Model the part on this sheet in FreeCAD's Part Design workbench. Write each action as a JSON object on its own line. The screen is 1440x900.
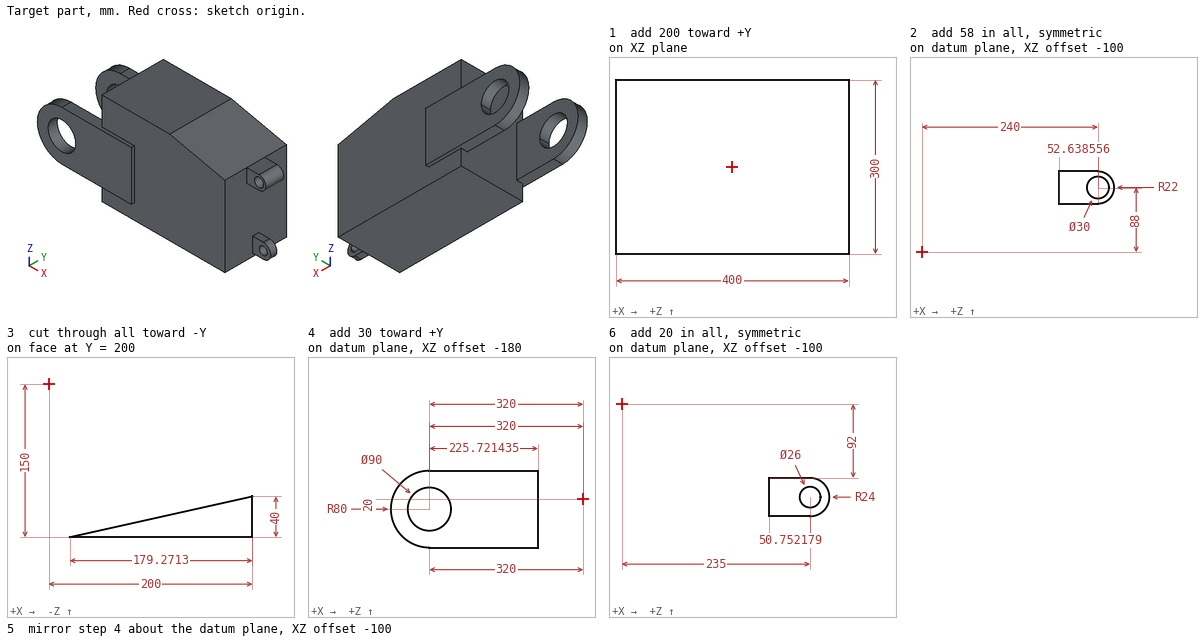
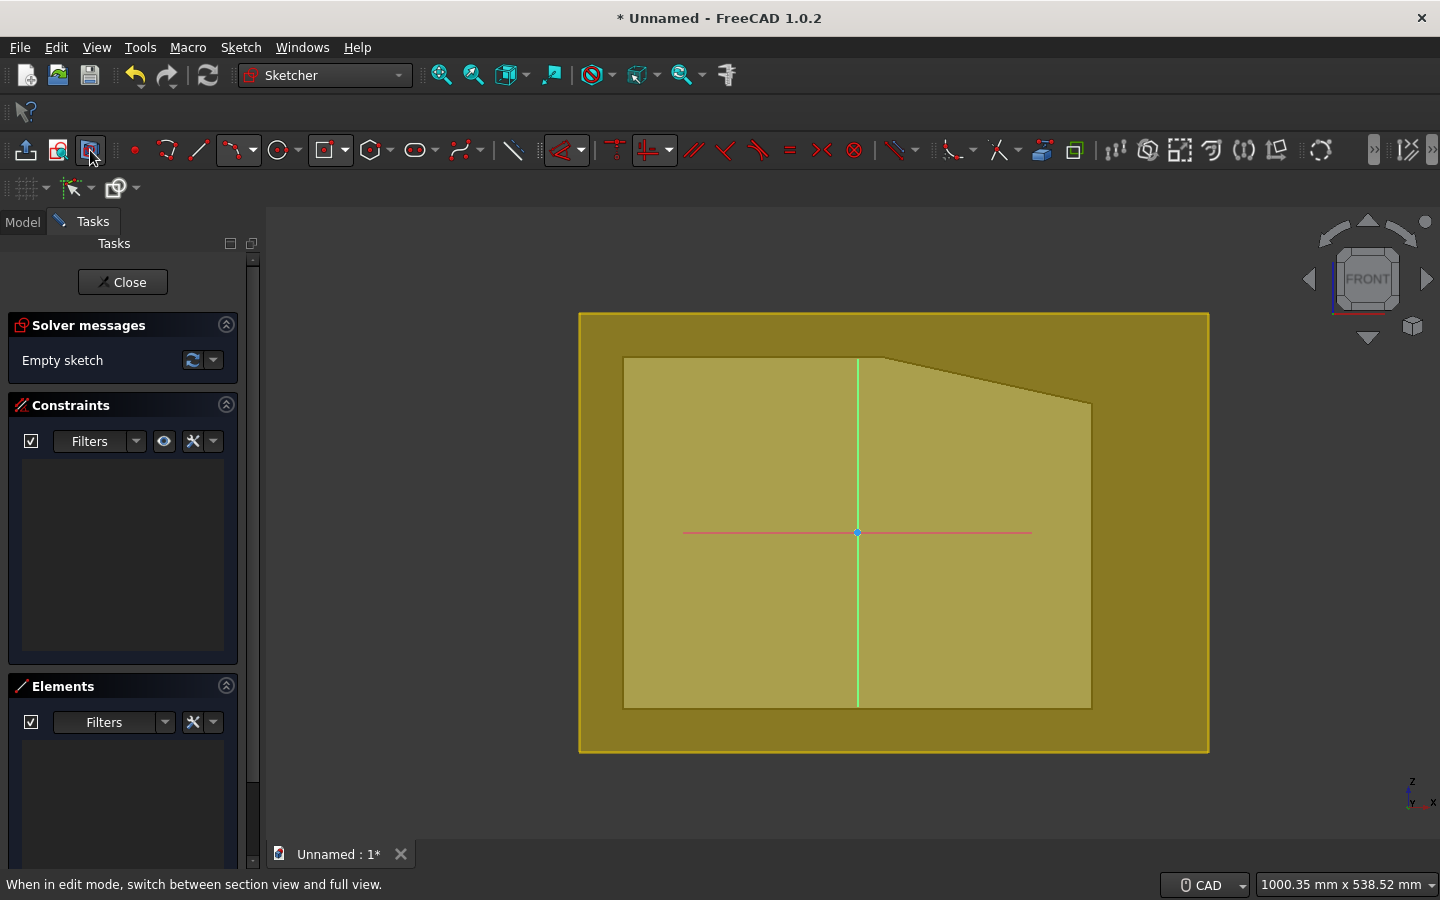
{"action": "scroll", "coordinate": [295, 624], "scroll_direction": "up", "scroll_amount": 2}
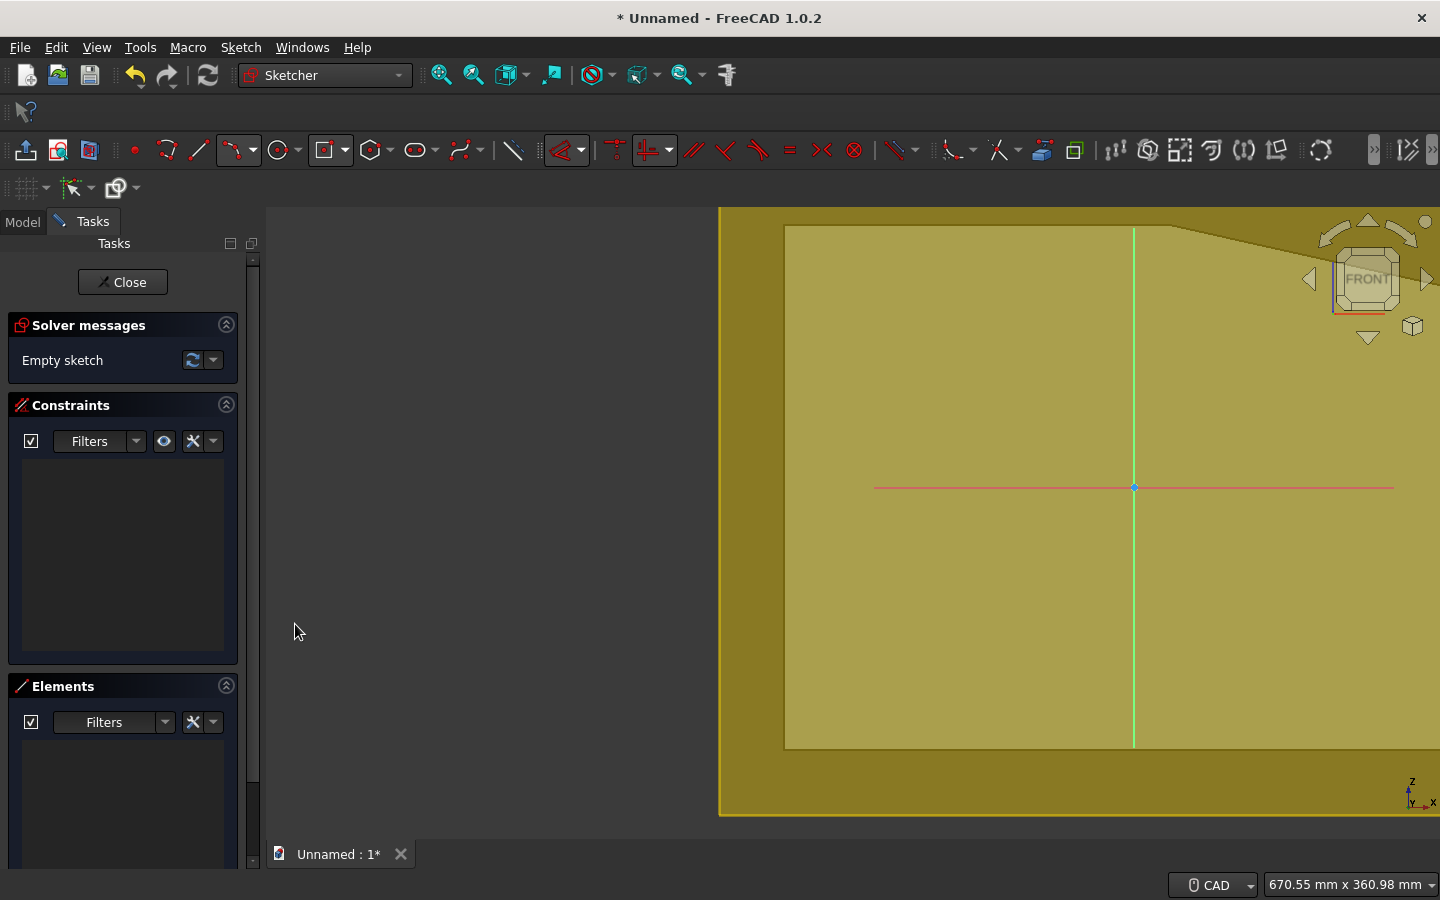
{"action": "left_click", "coordinate": [168, 150]}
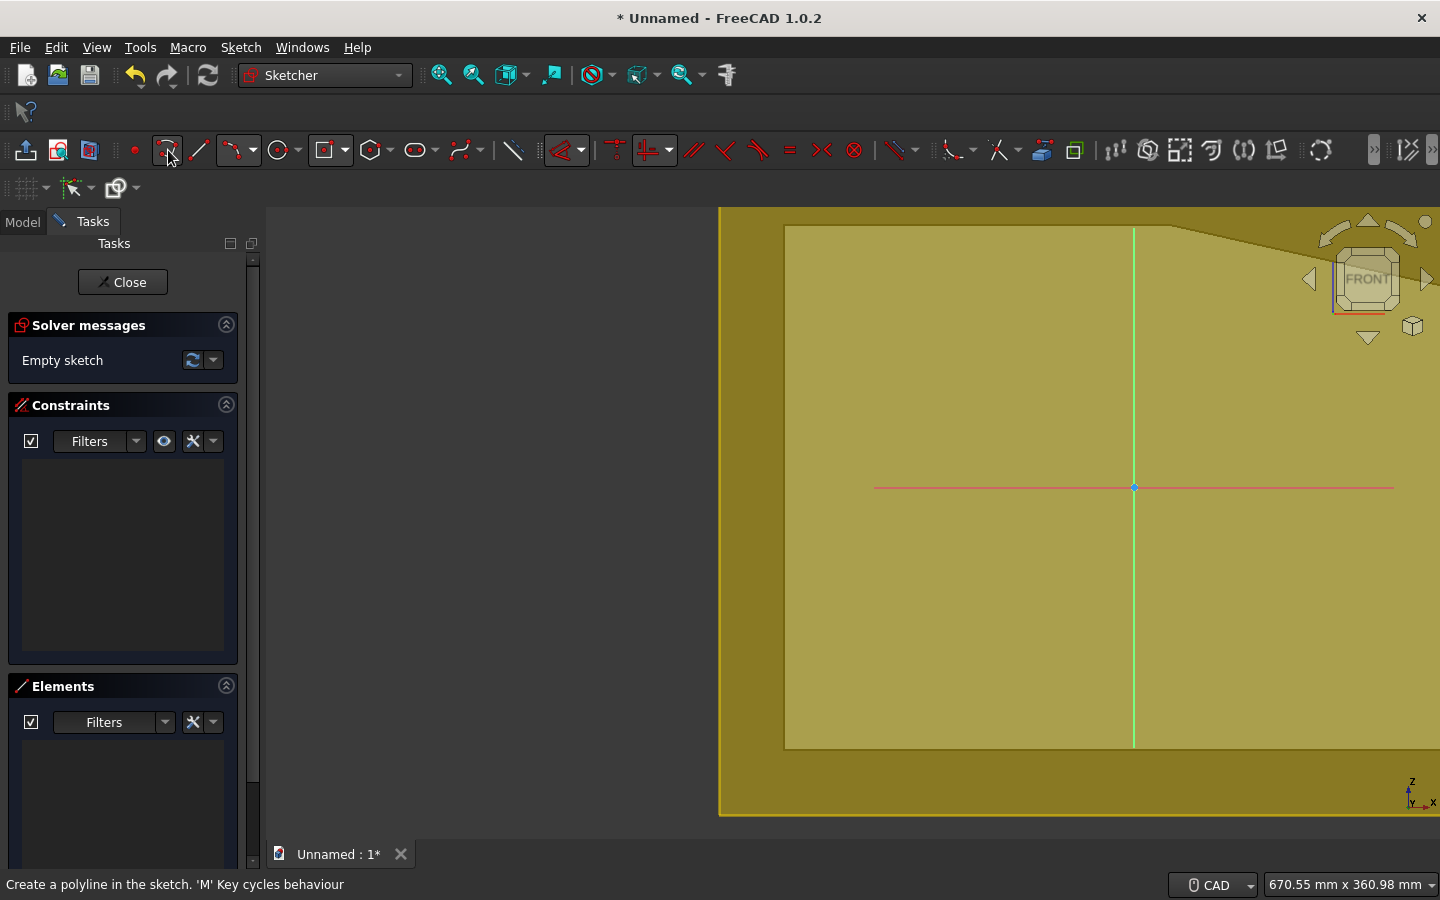
{"action": "left_click", "coordinate": [574, 383]}
{"action": "left_click", "coordinate": [969, 383]}
{"action": "left_click", "coordinate": [969, 663]}
{"action": "left_click", "coordinate": [574, 663]}
{"action": "right_click", "coordinate": [574, 663]}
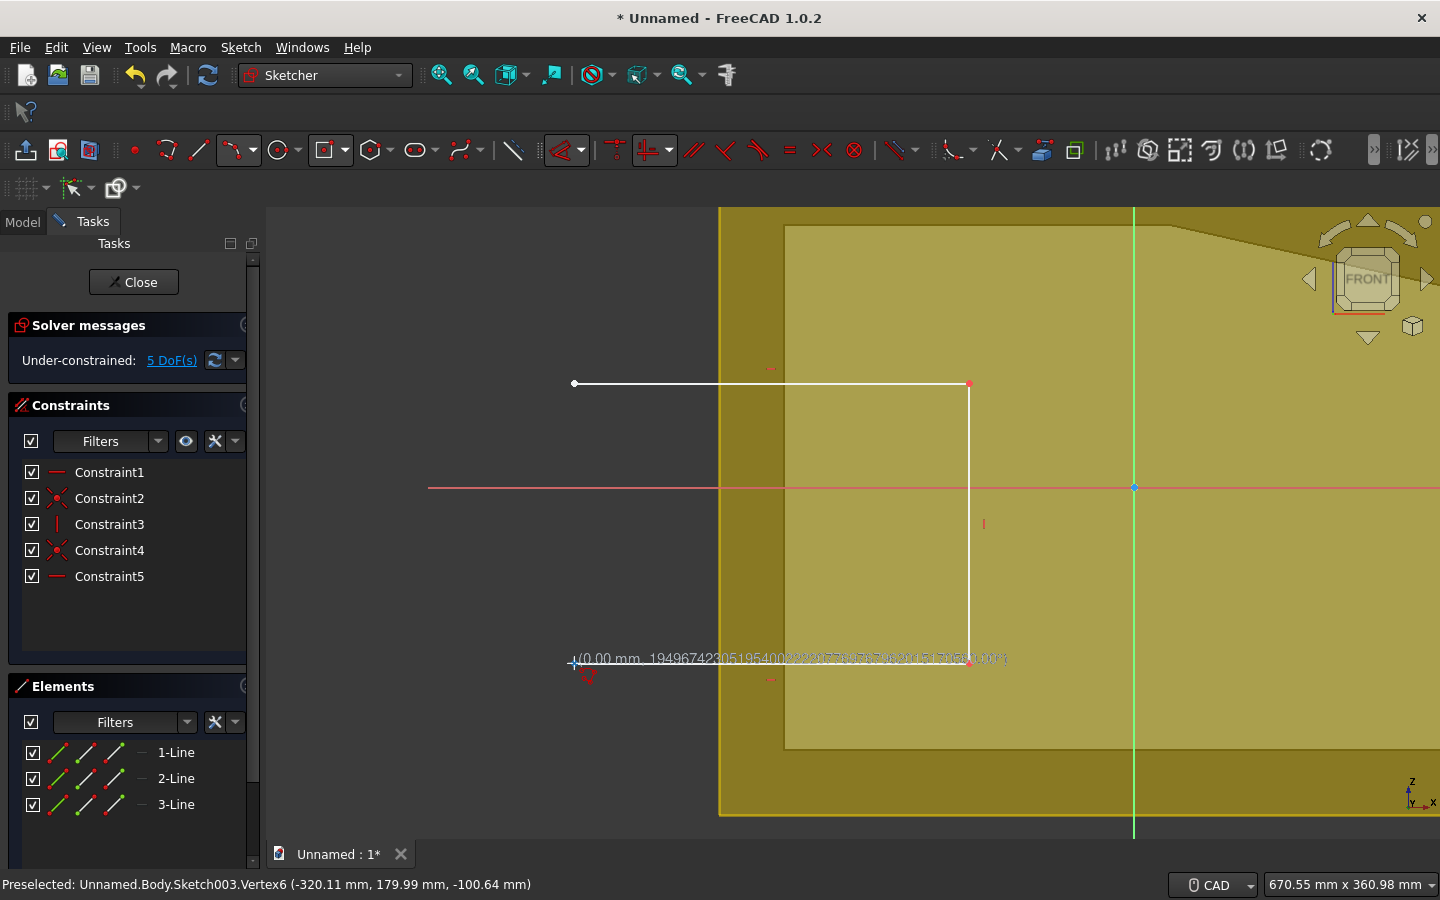
{"action": "left_click", "coordinate": [232, 150]}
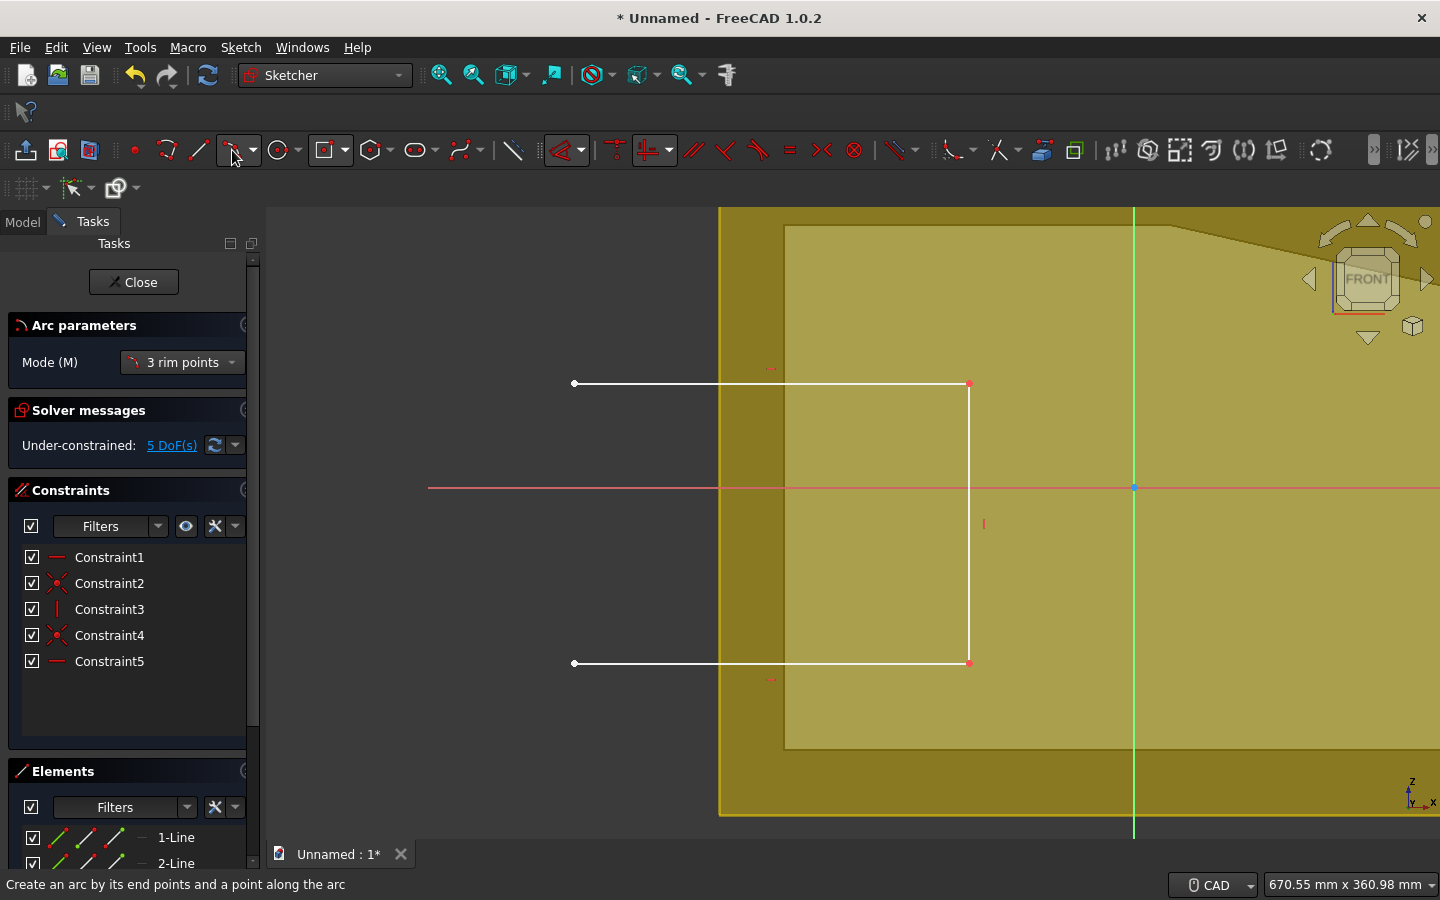
{"action": "left_click", "coordinate": [574, 664]}
{"action": "left_click", "coordinate": [574, 384]}
{"action": "left_click", "coordinate": [434, 523]}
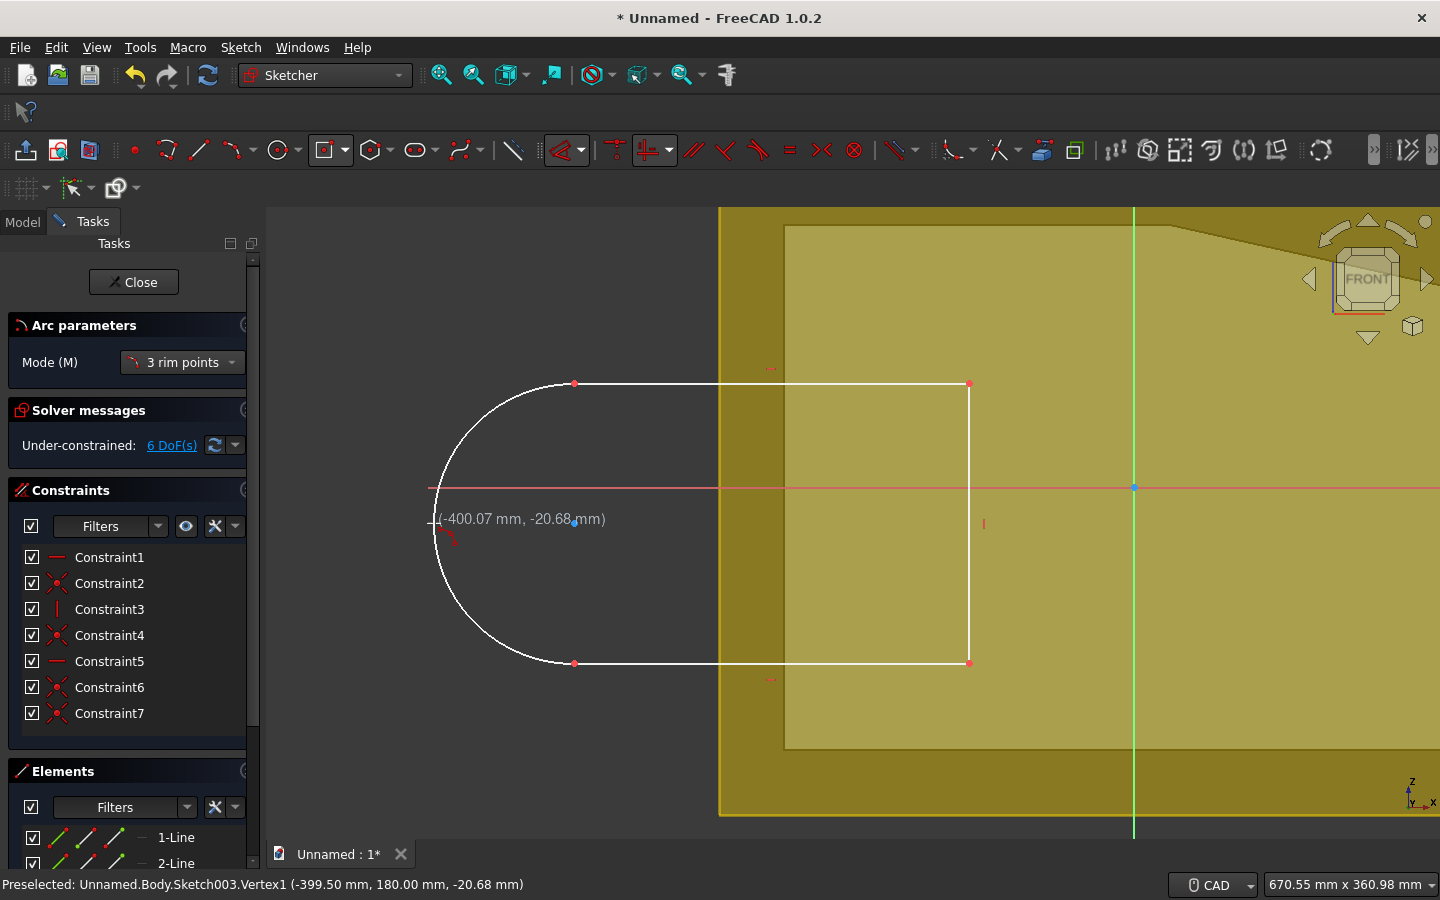
{"action": "left_click", "coordinate": [278, 150]}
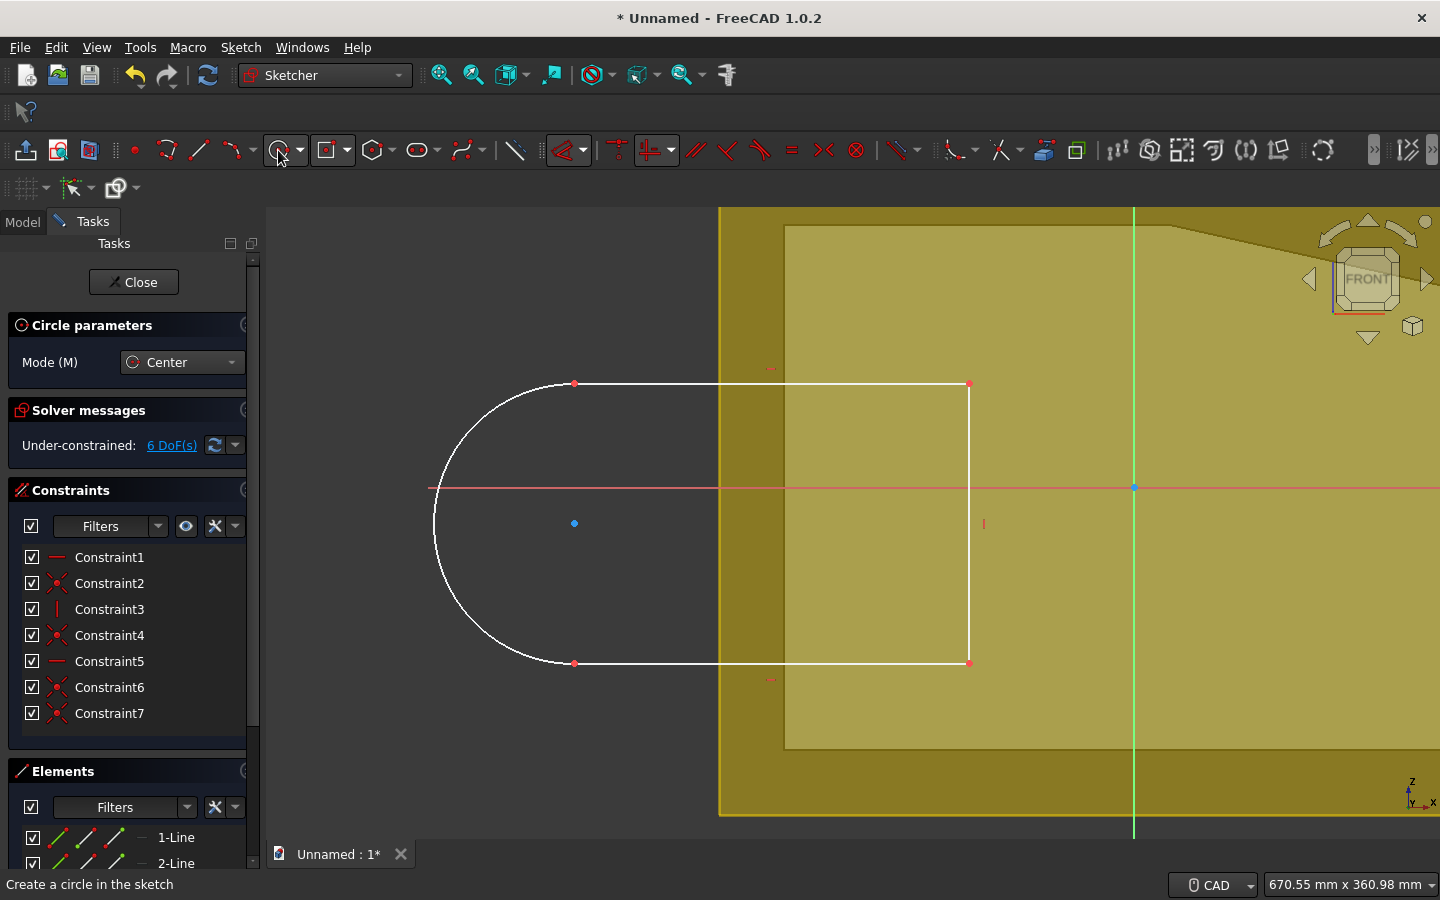
{"action": "left_click", "coordinate": [574, 523]}
{"action": "left_click", "coordinate": [630, 467]}
{"action": "key", "text": "Escape"}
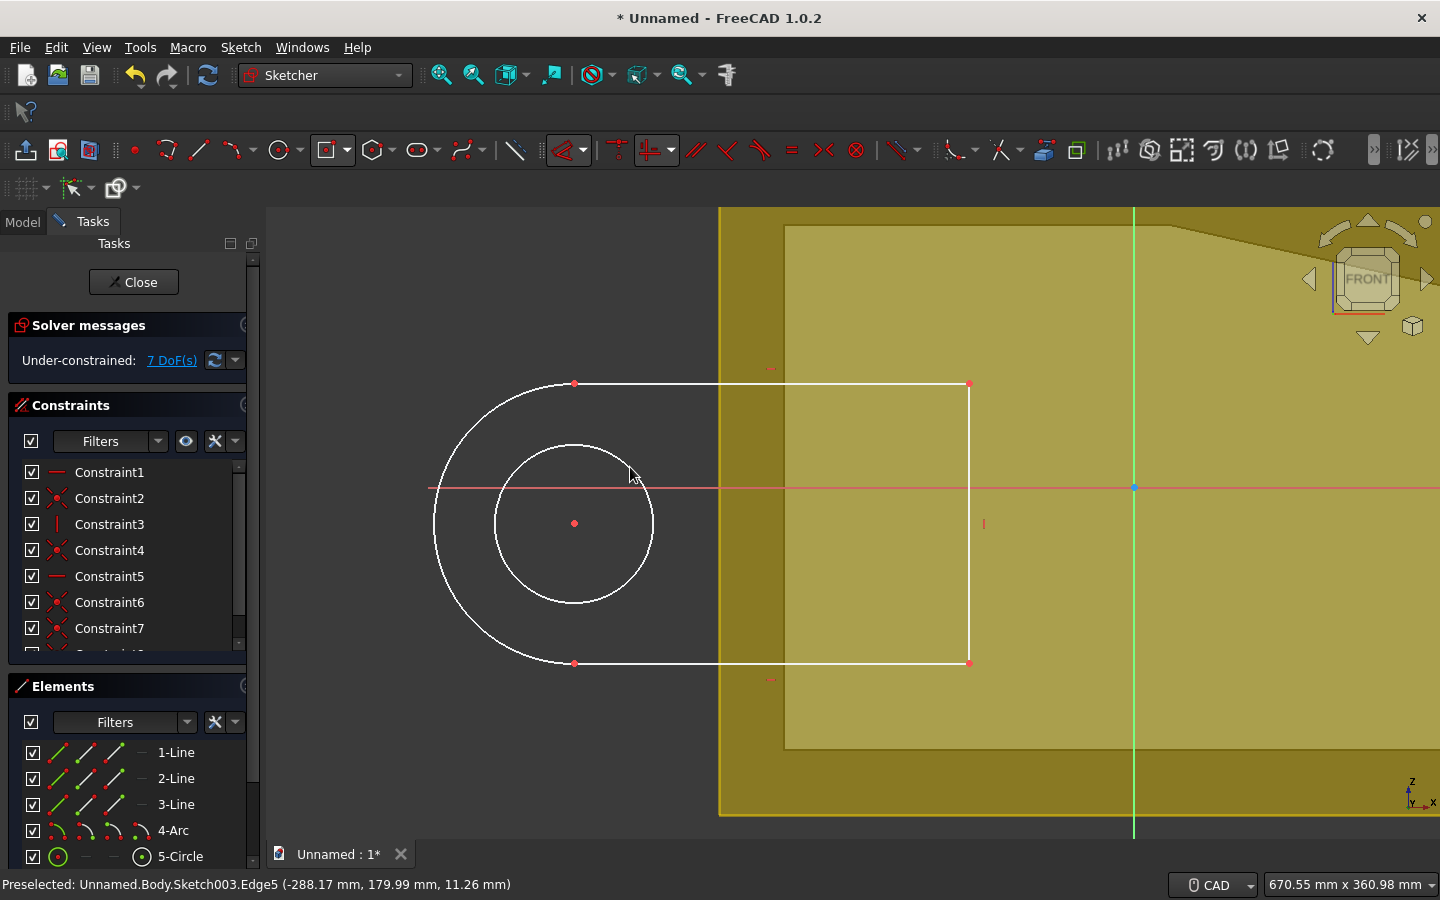
{"action": "left_click", "coordinate": [461, 442]}